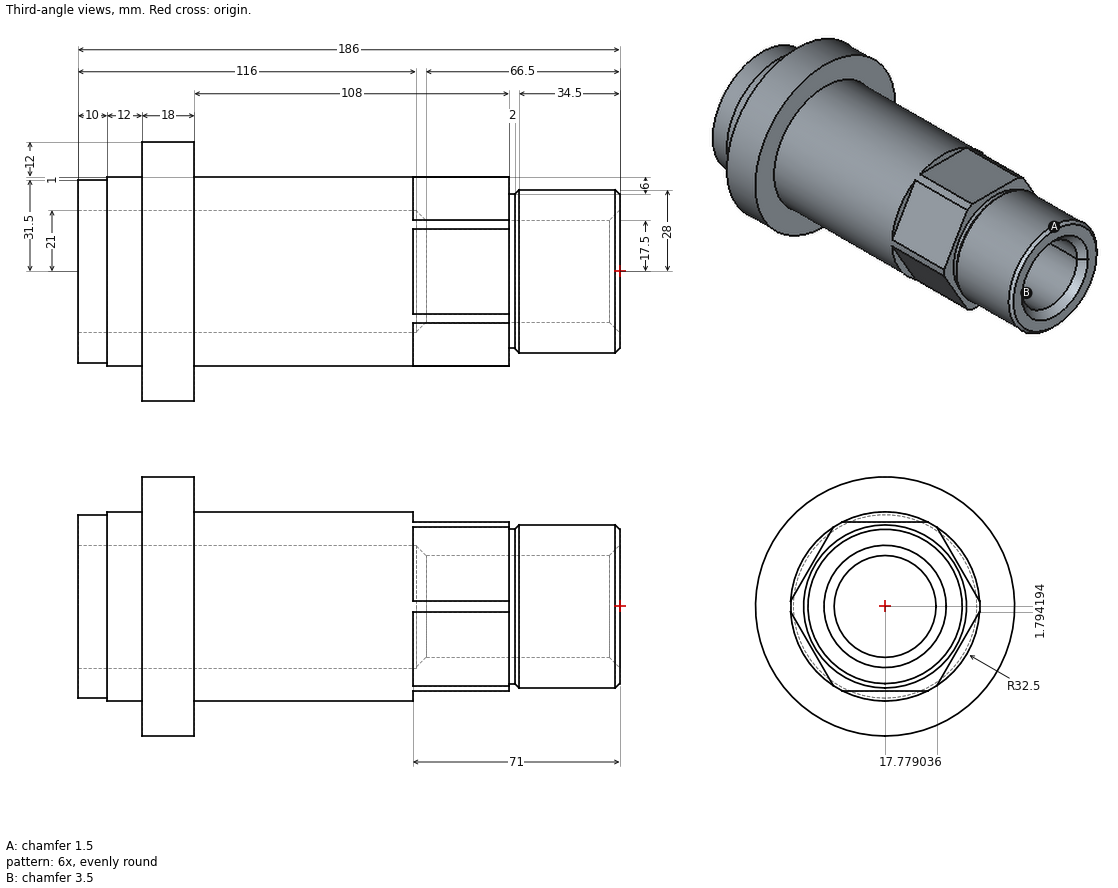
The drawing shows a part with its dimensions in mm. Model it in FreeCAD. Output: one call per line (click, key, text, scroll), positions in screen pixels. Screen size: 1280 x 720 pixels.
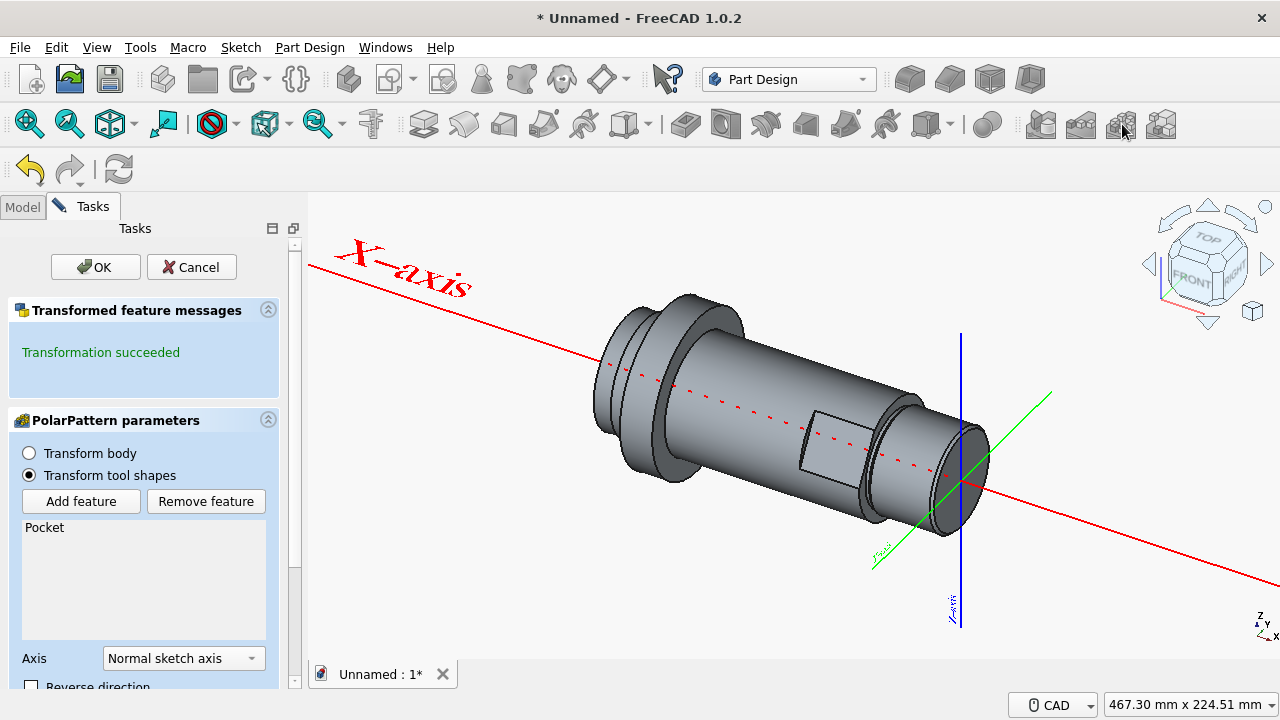
click(184, 658)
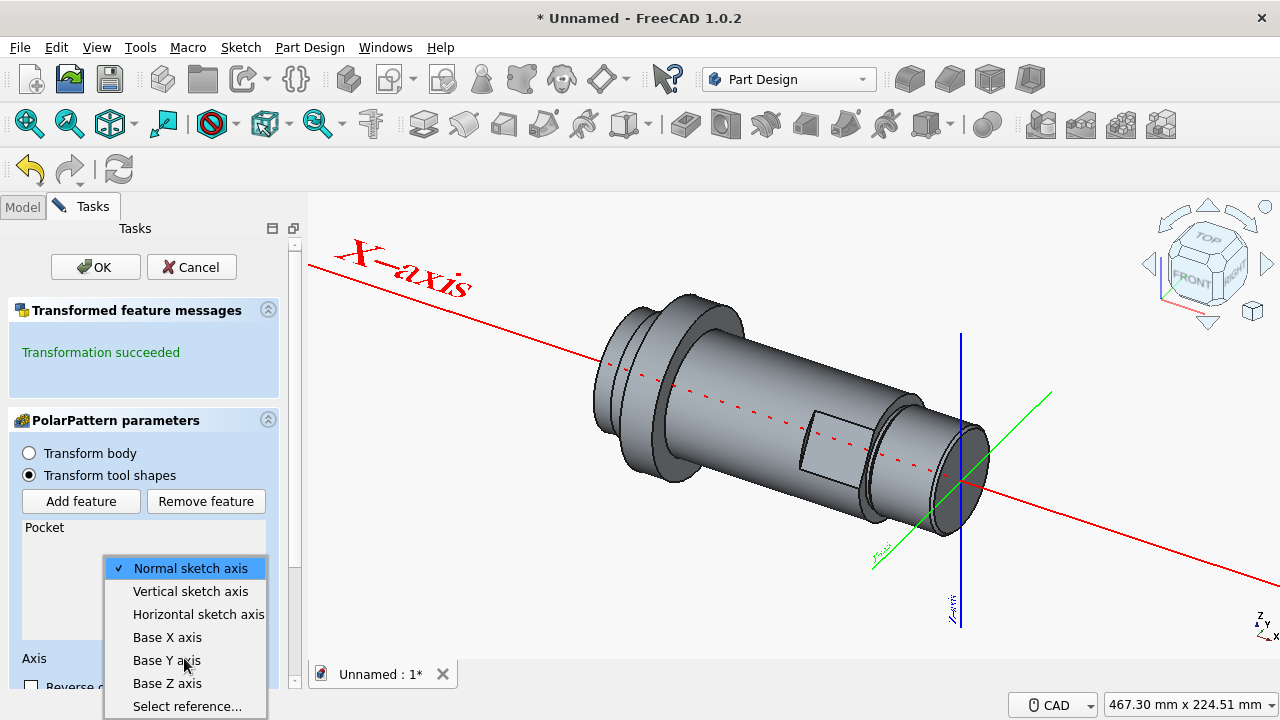
click(184, 638)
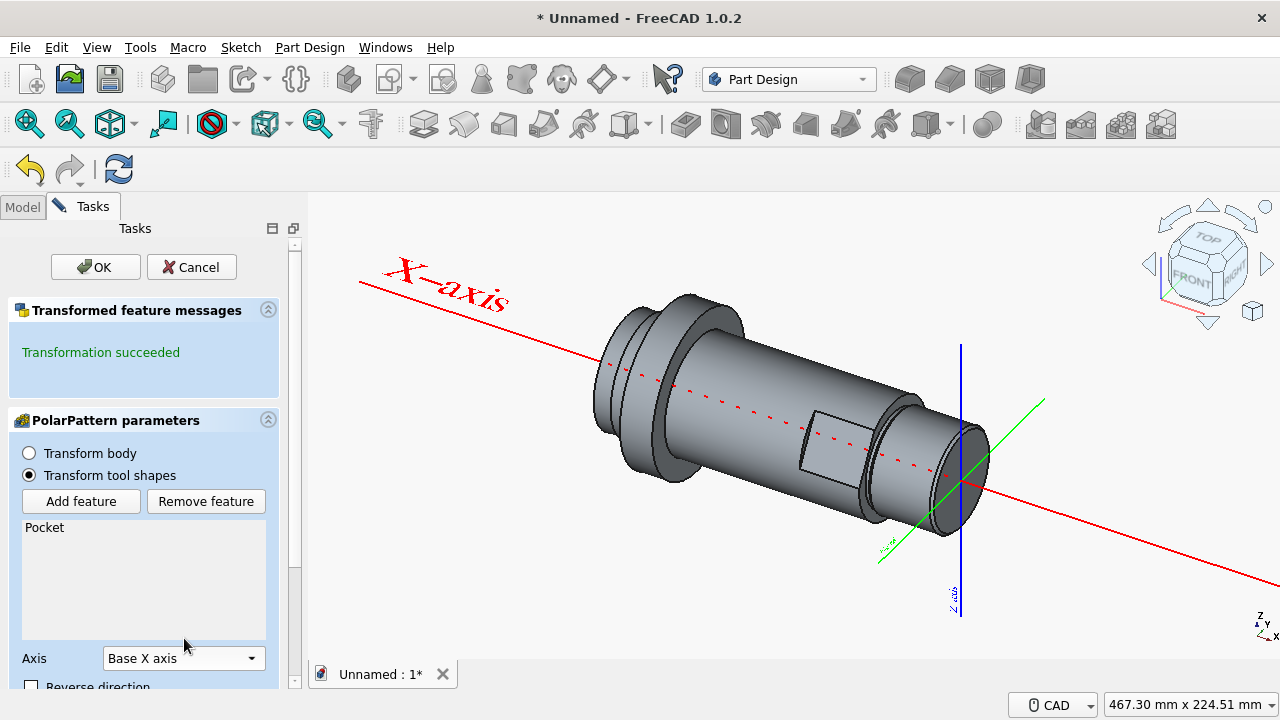
scroll(295, 463, down, 3)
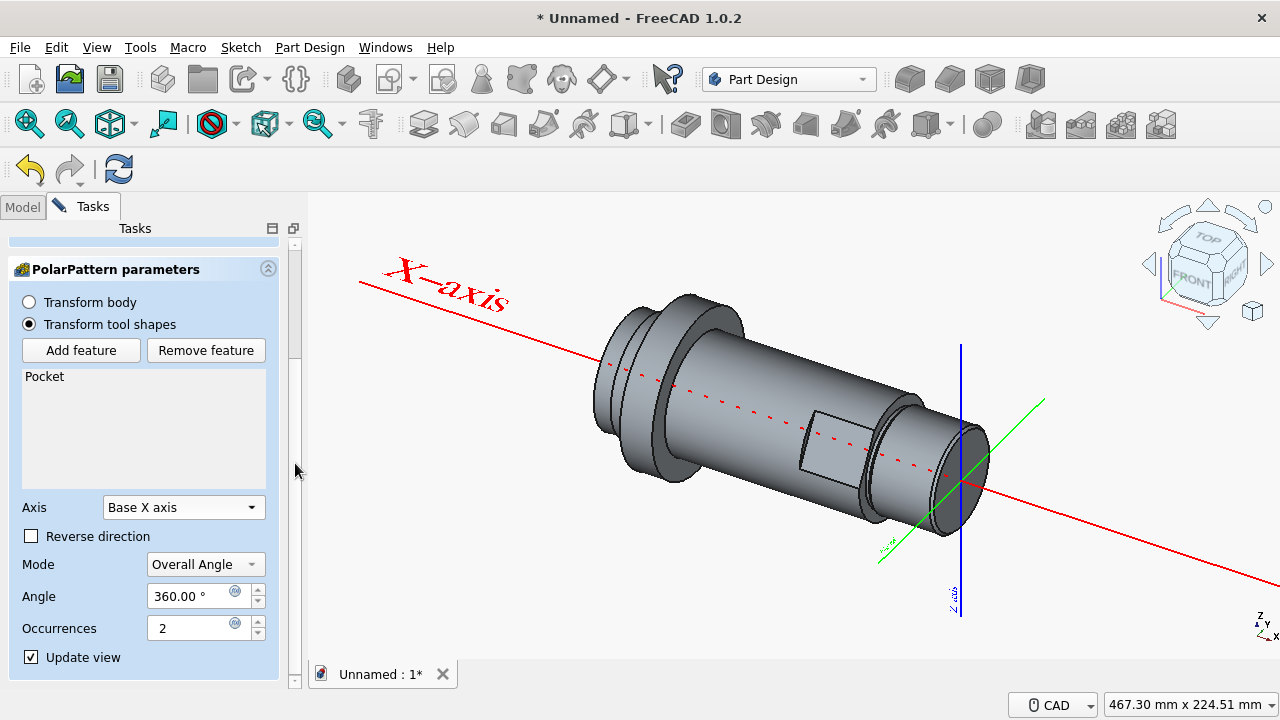
triple_click(198, 628)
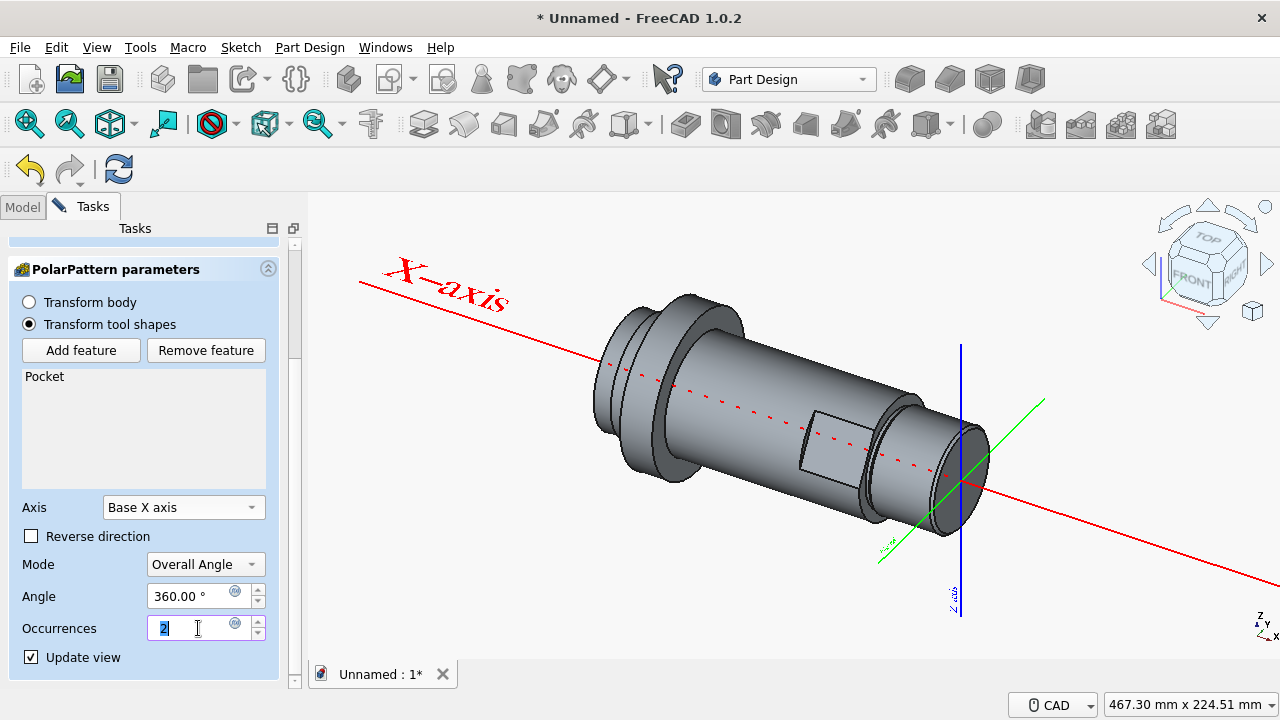
text(6)
key(Tab)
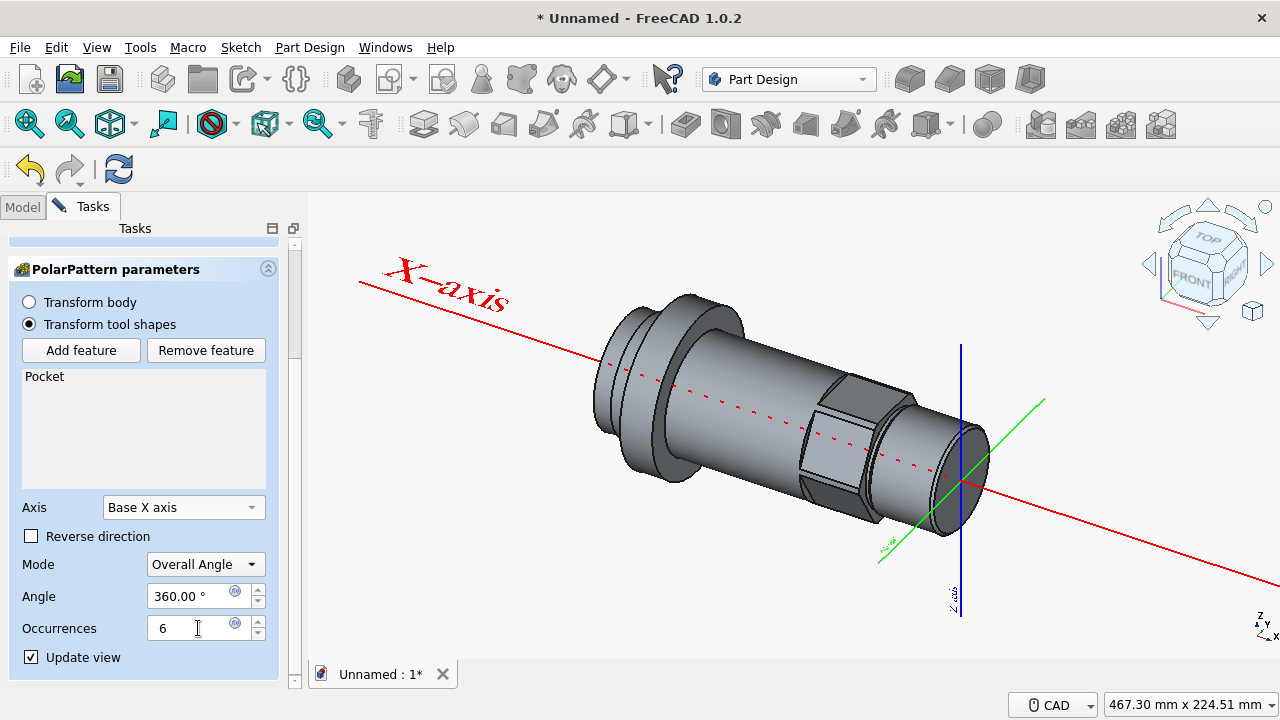
scroll(295, 463, up, 4)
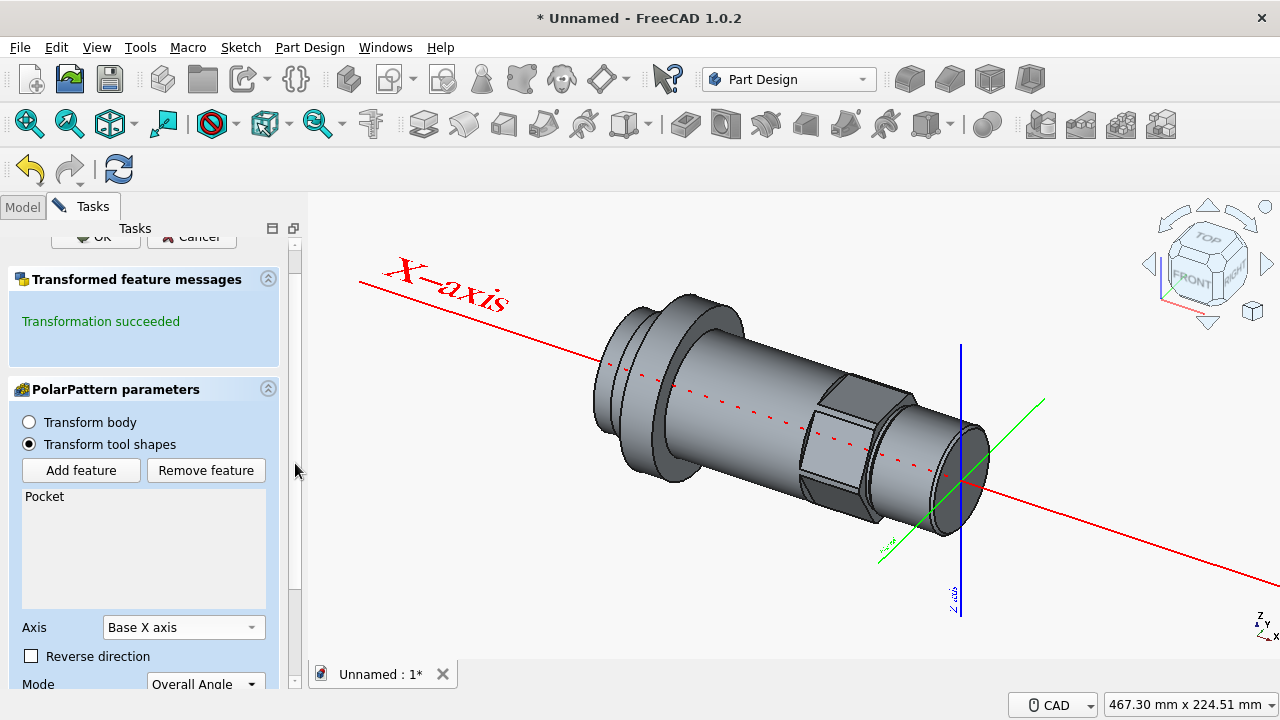
click(96, 267)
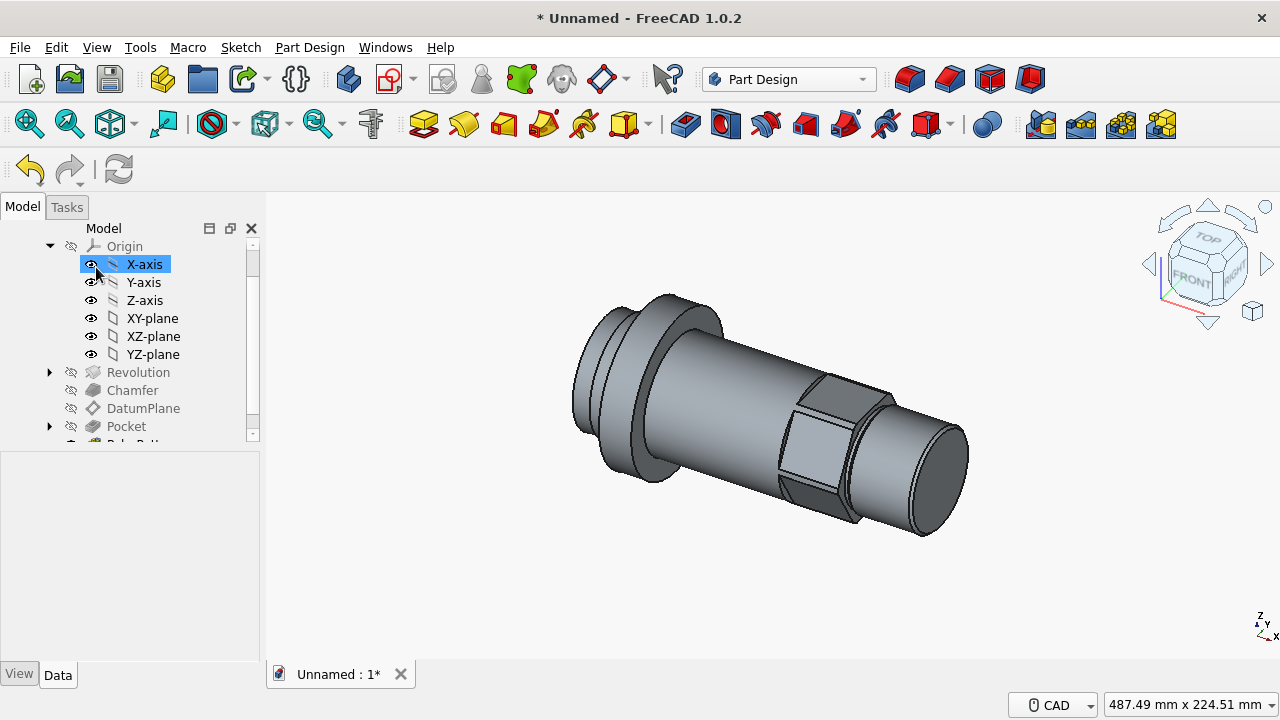
click(390, 80)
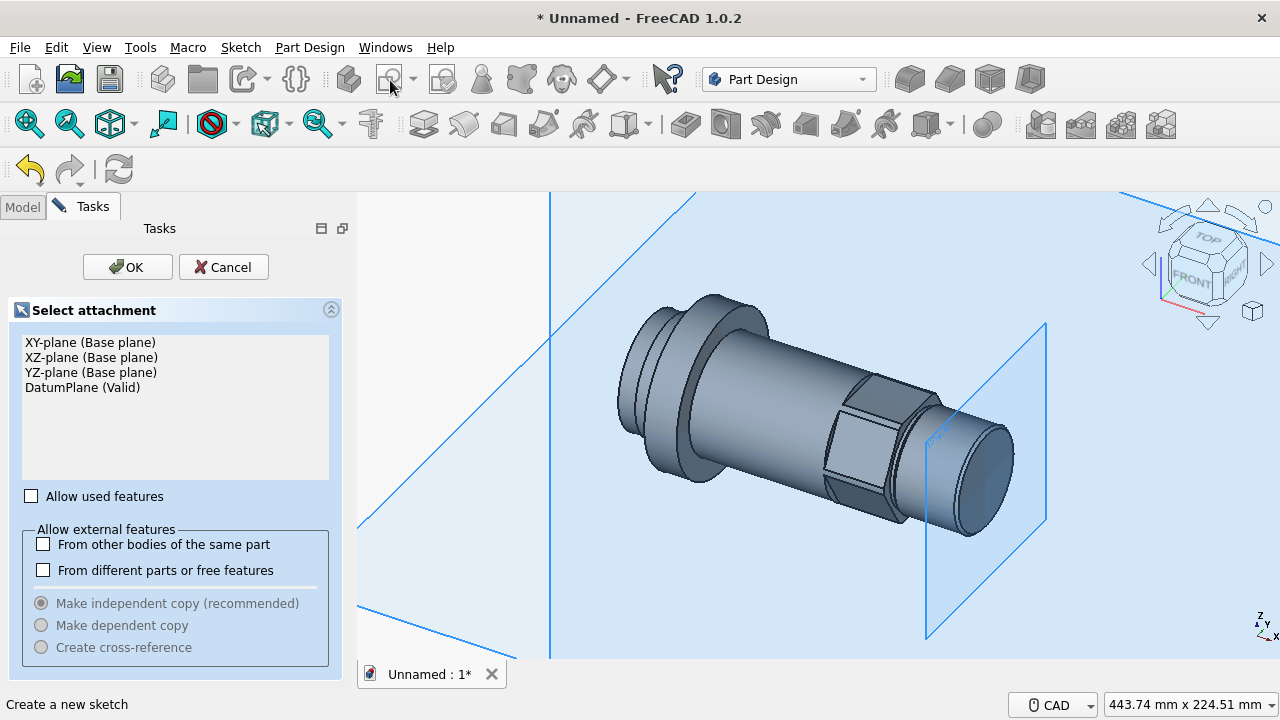
click(82, 342)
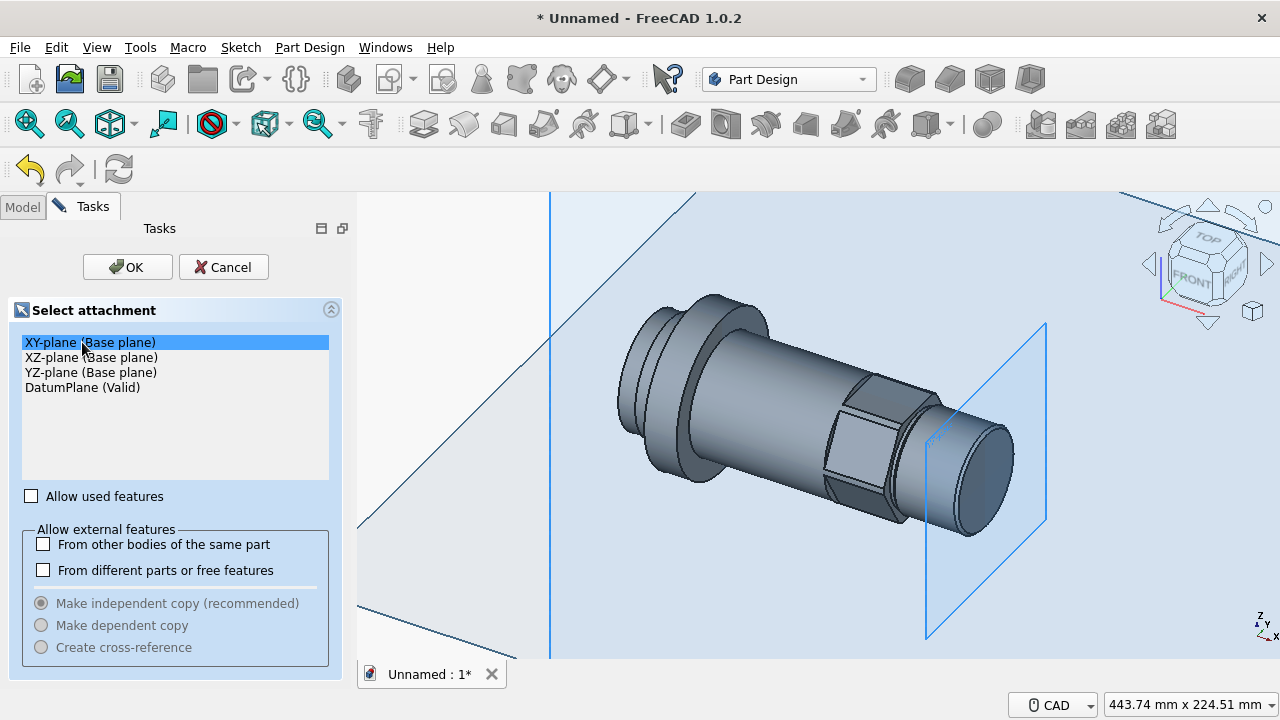
click(128, 267)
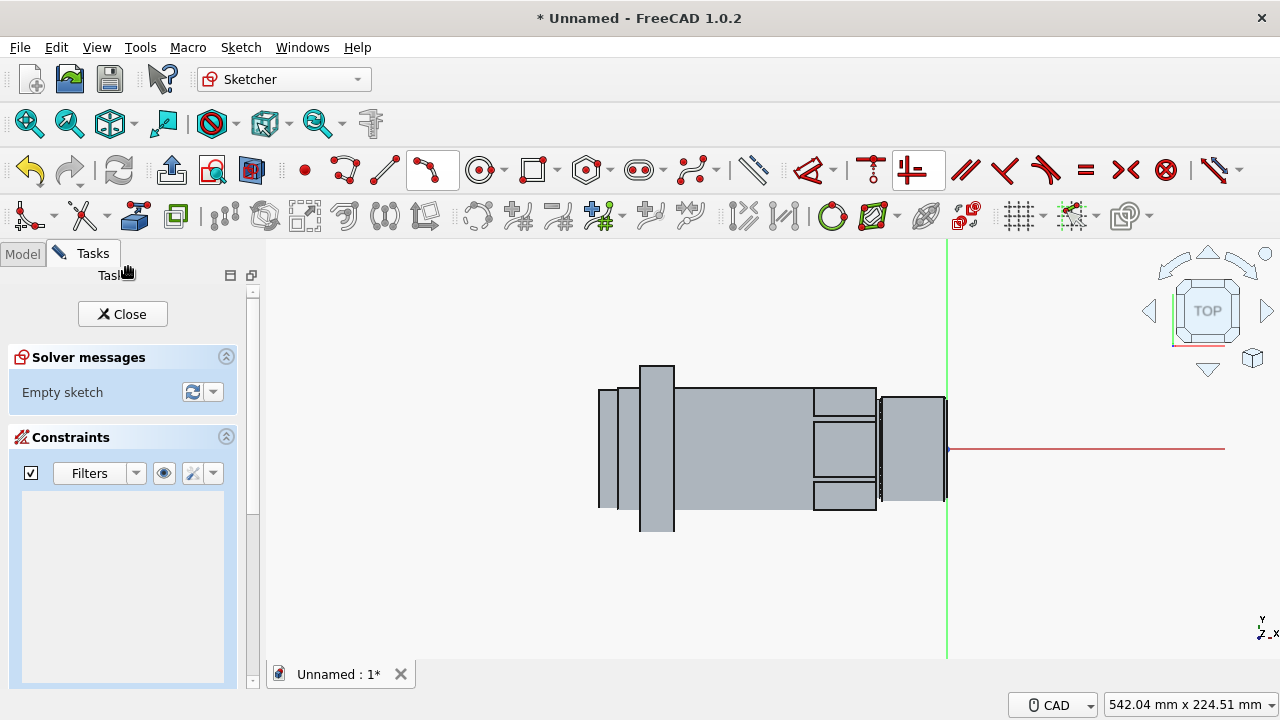
click(252, 170)